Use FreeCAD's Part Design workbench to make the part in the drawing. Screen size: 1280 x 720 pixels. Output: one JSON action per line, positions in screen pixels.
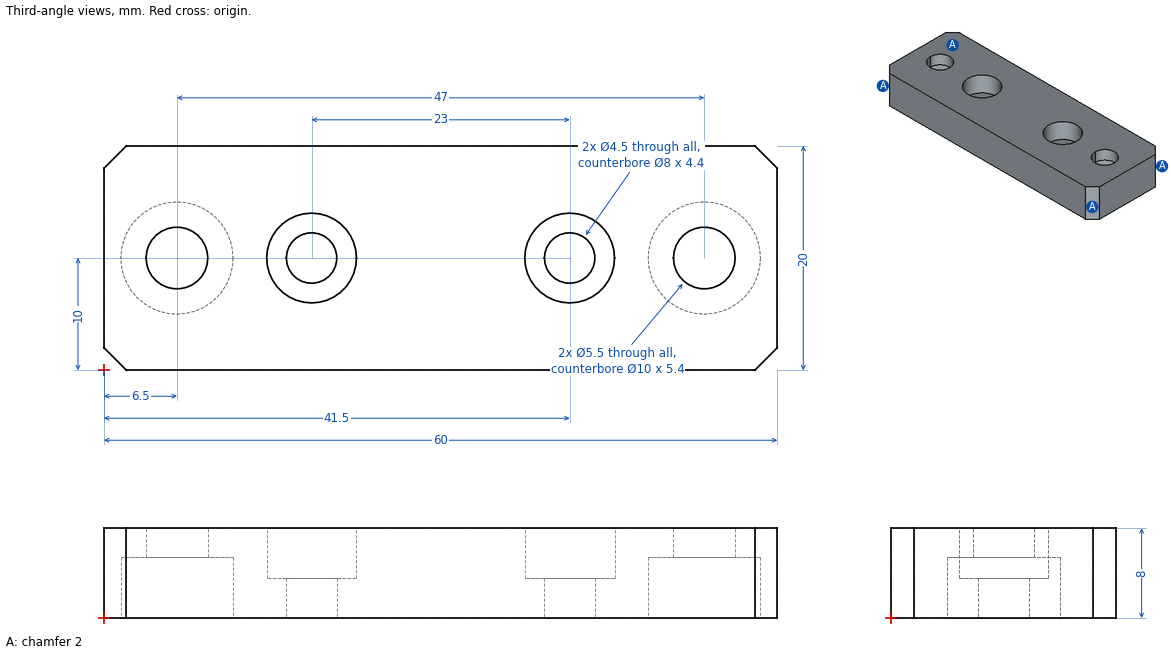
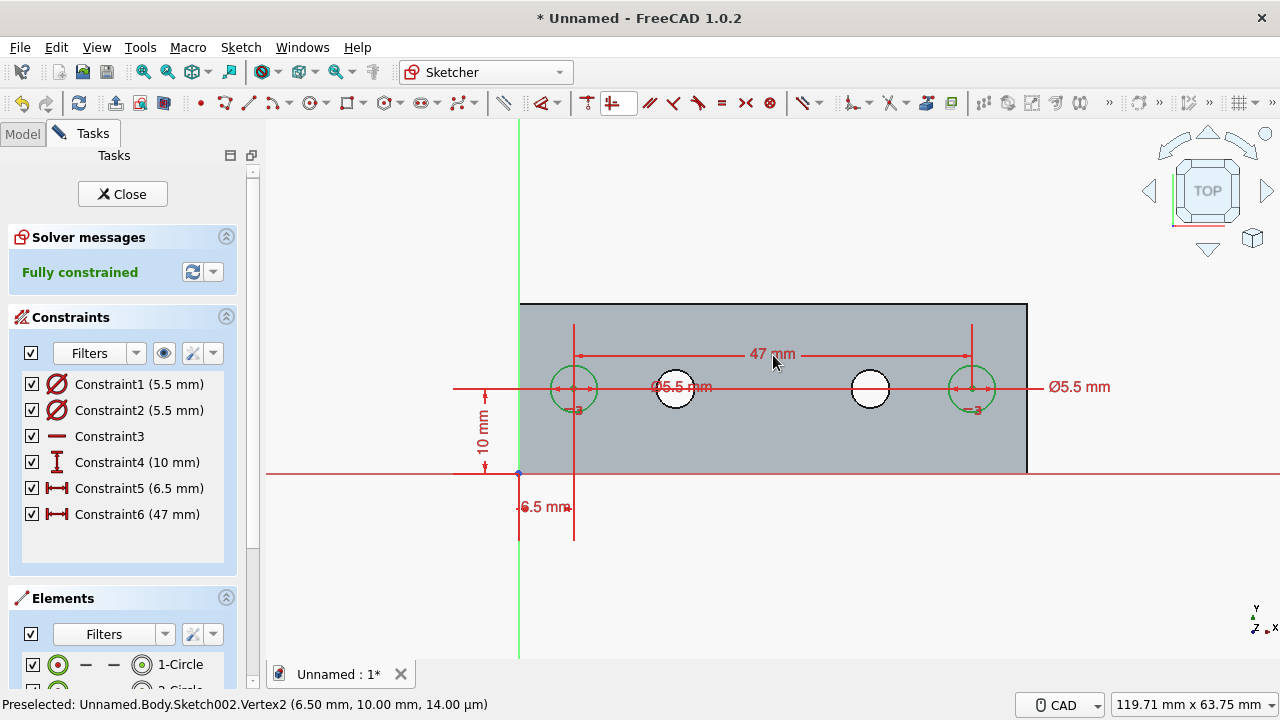
{"action": "left_click", "coordinate": [123, 194]}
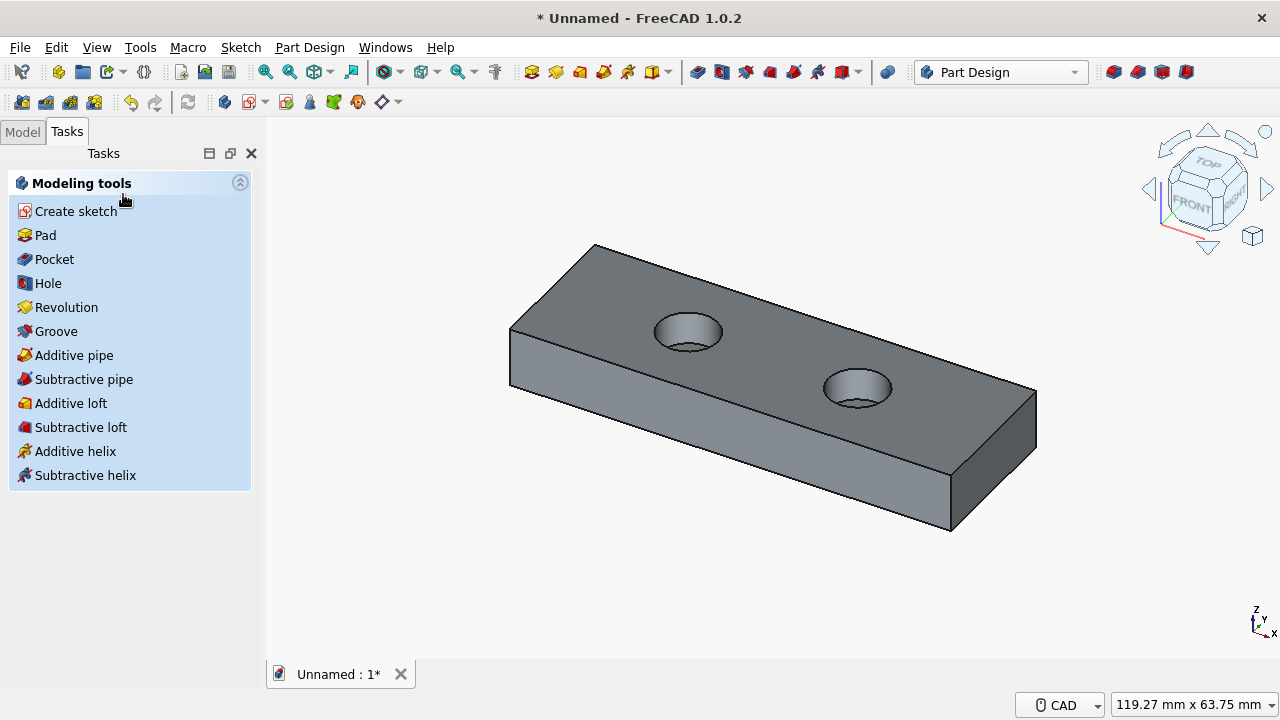
{"action": "left_click", "coordinate": [722, 72]}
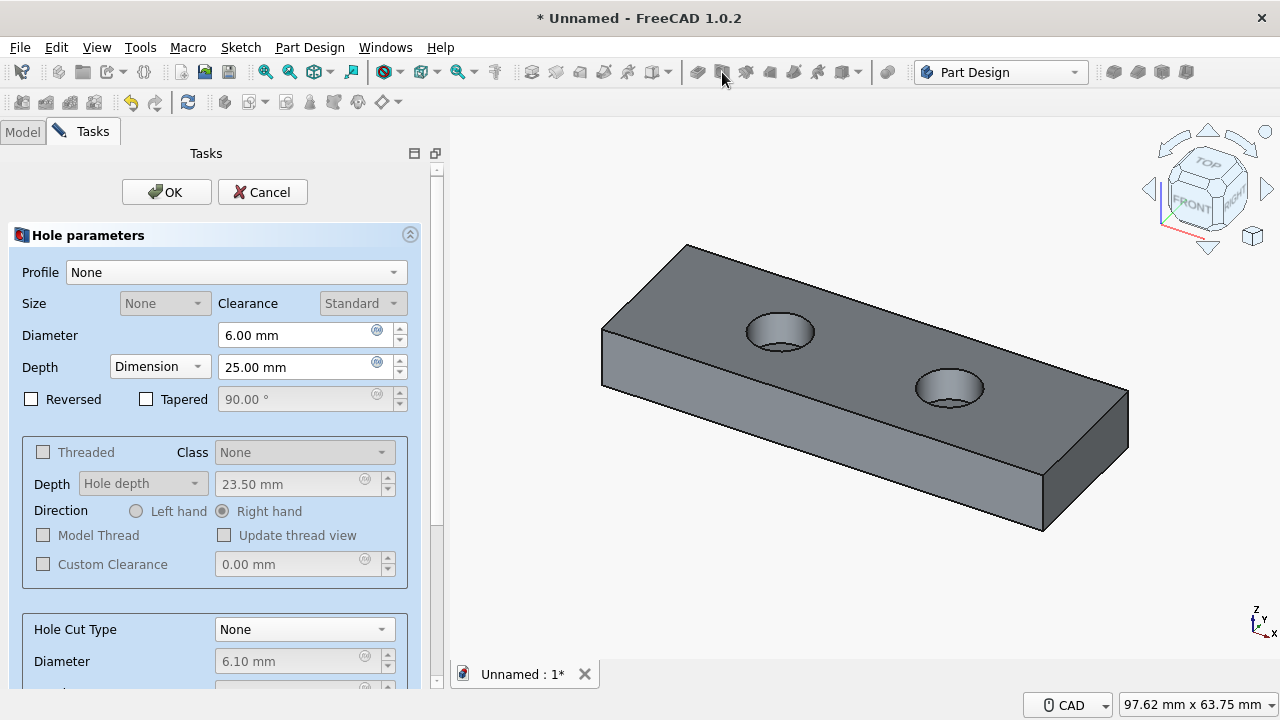
{"action": "triple_click", "coordinate": [305, 335]}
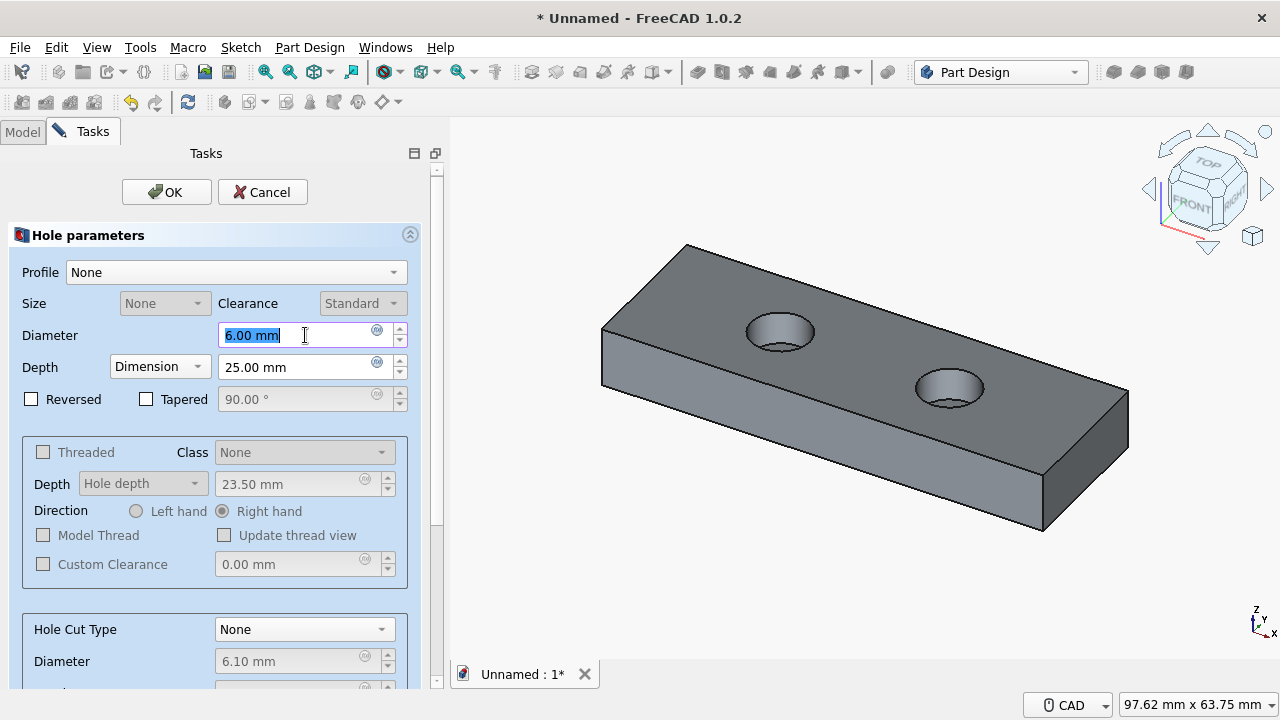
{"action": "type", "text": "5.5"}
{"action": "key", "text": "Tab"}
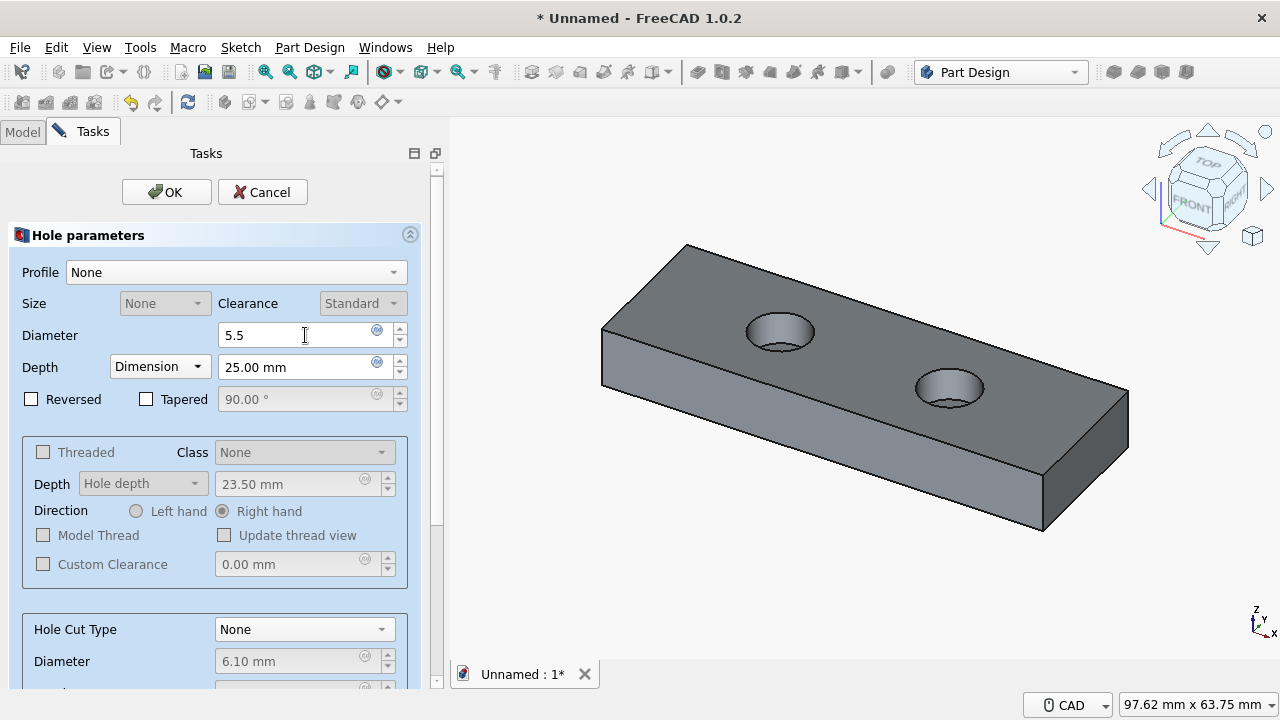
{"action": "left_click", "coordinate": [161, 366]}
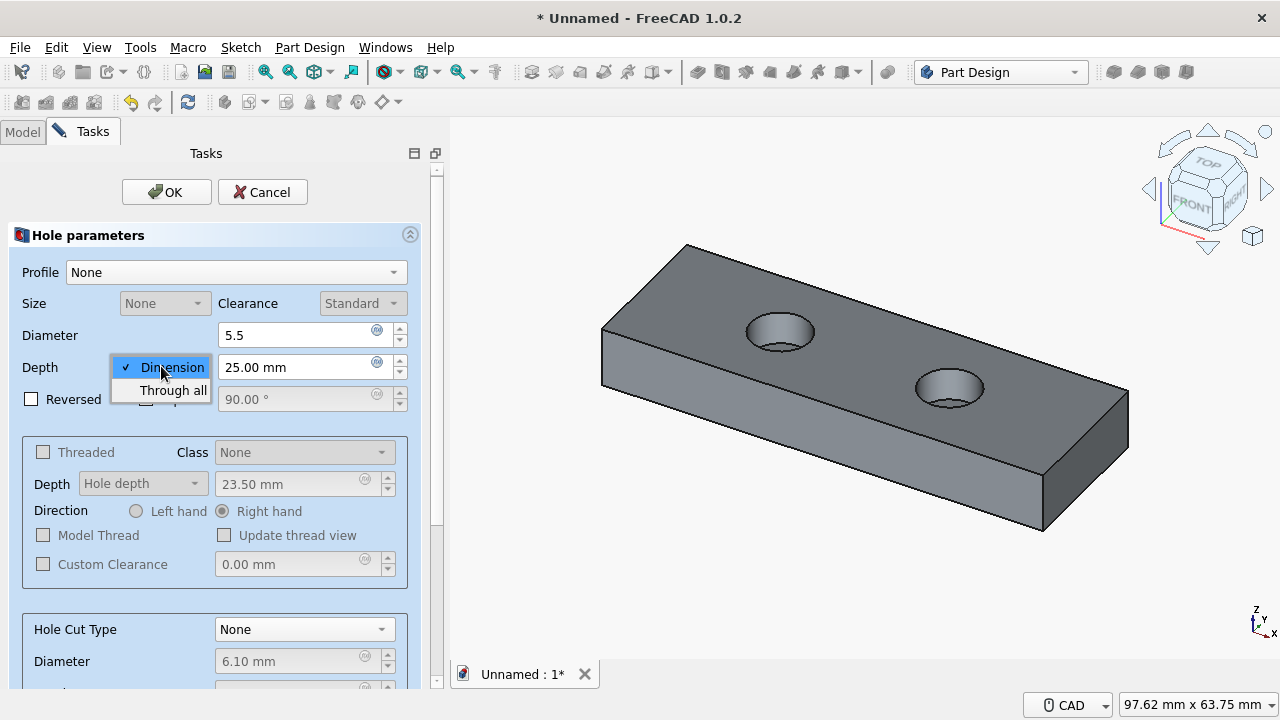
{"action": "left_click", "coordinate": [160, 390]}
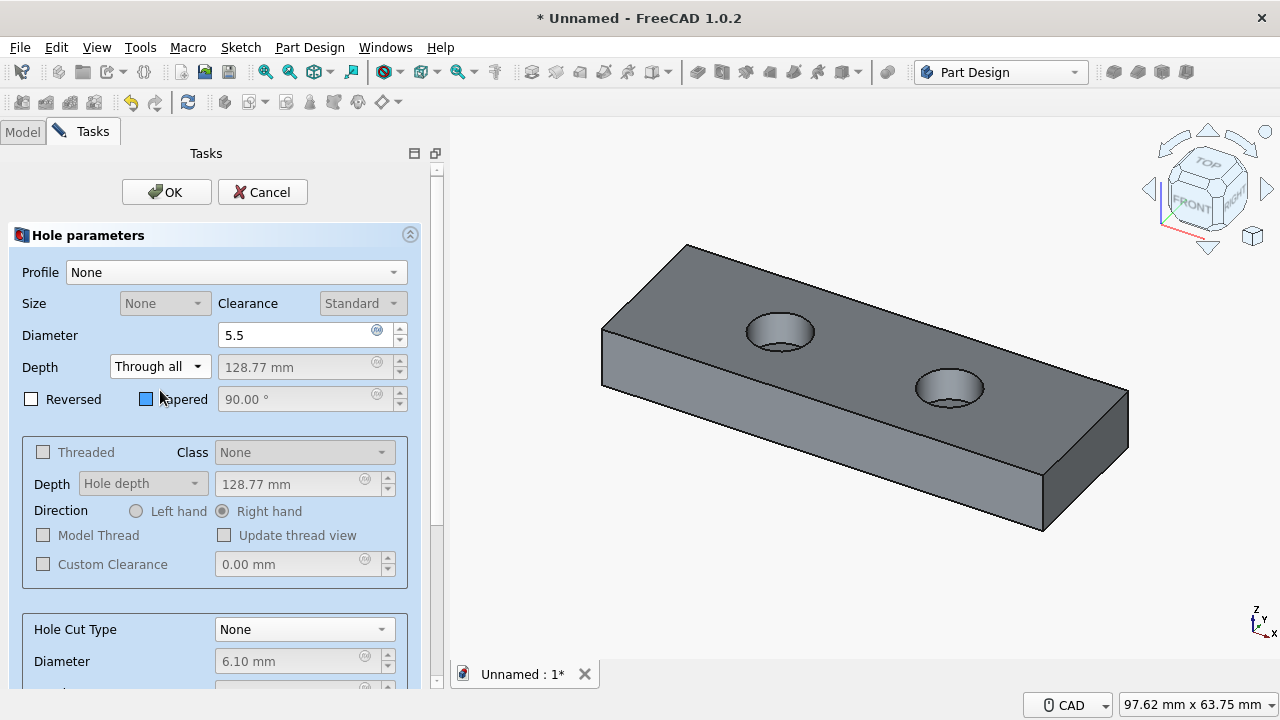
{"action": "left_click", "coordinate": [30, 399]}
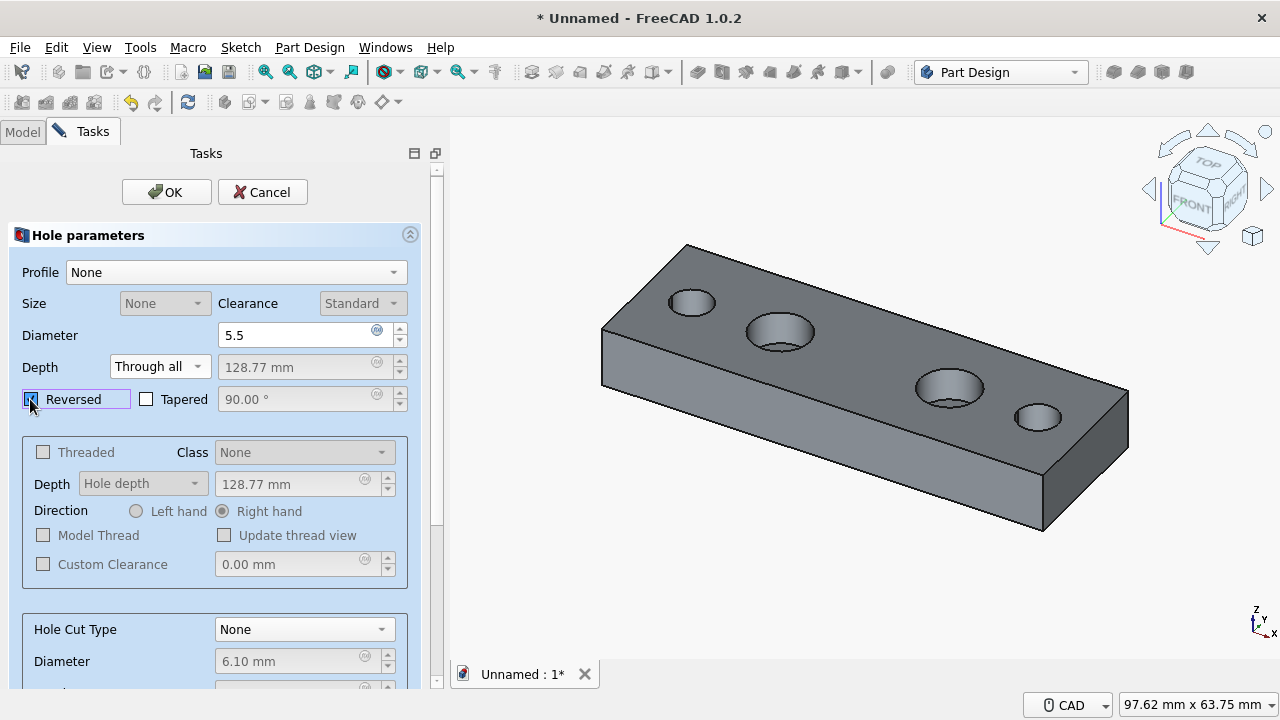
{"action": "left_click", "coordinate": [306, 630]}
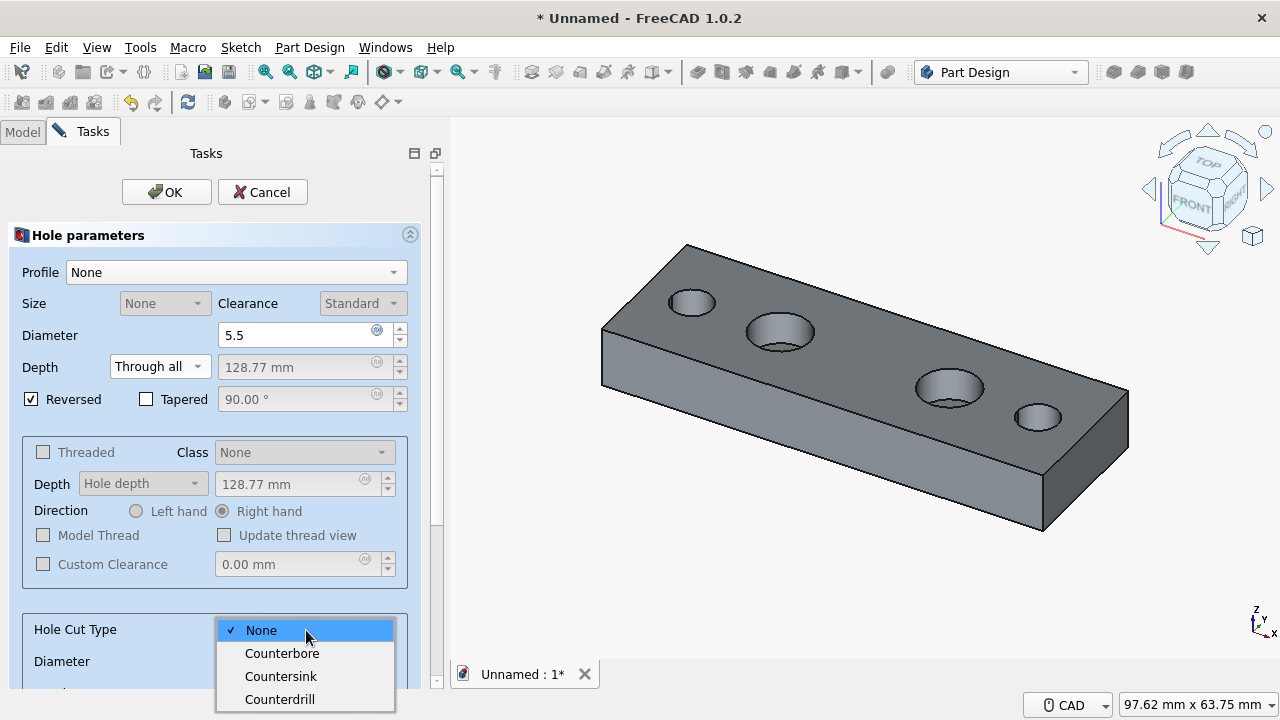
{"action": "left_click", "coordinate": [304, 654]}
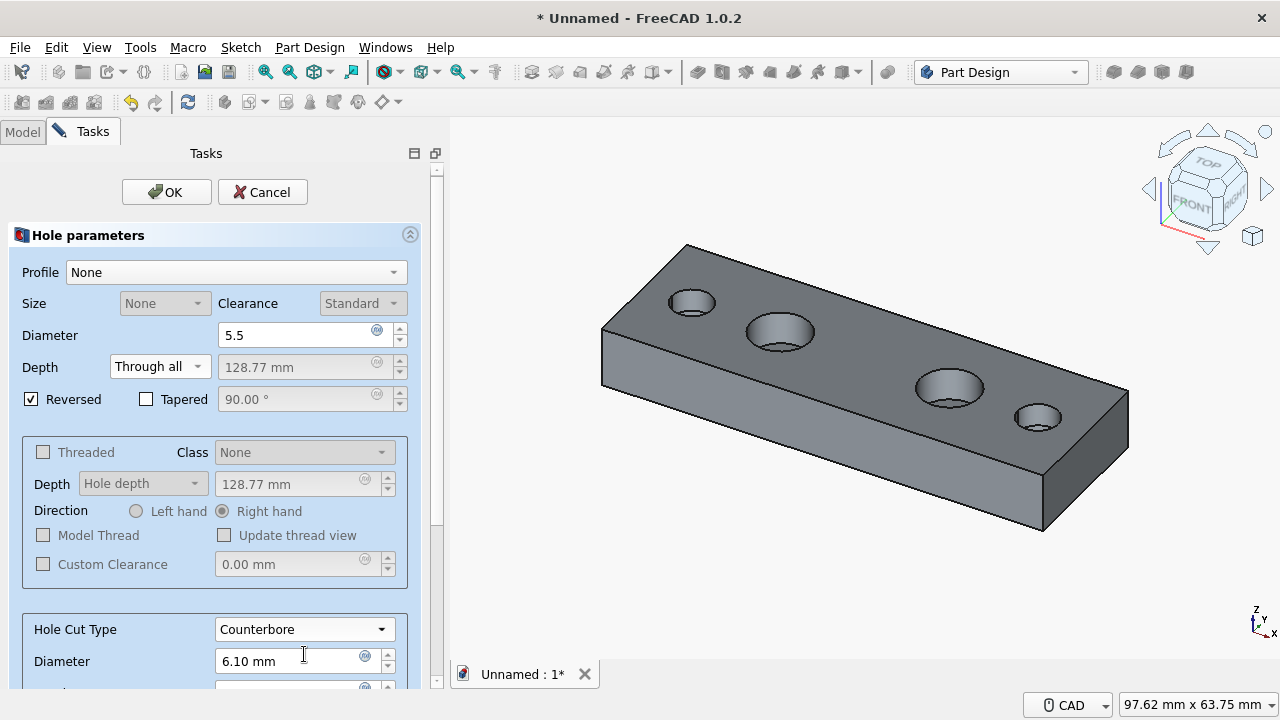
{"action": "triple_click", "coordinate": [298, 661]}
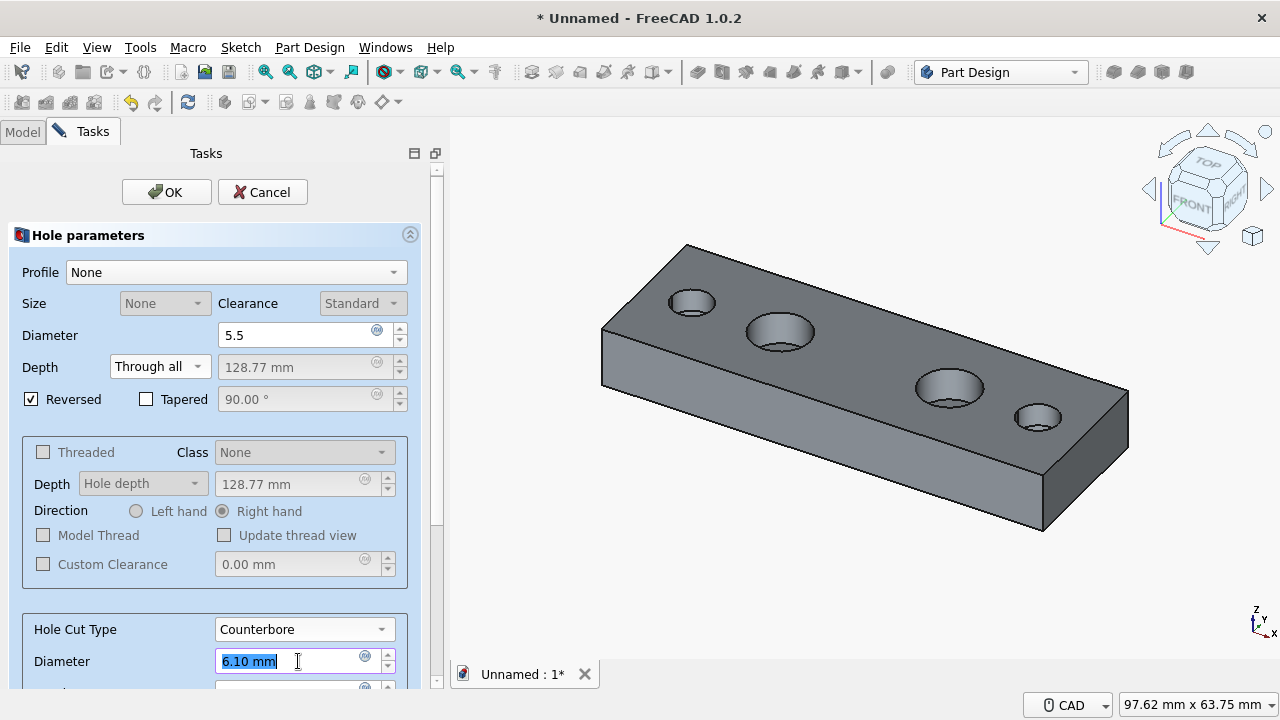
{"action": "type", "text": "10"}
{"action": "key", "text": "Tab"}